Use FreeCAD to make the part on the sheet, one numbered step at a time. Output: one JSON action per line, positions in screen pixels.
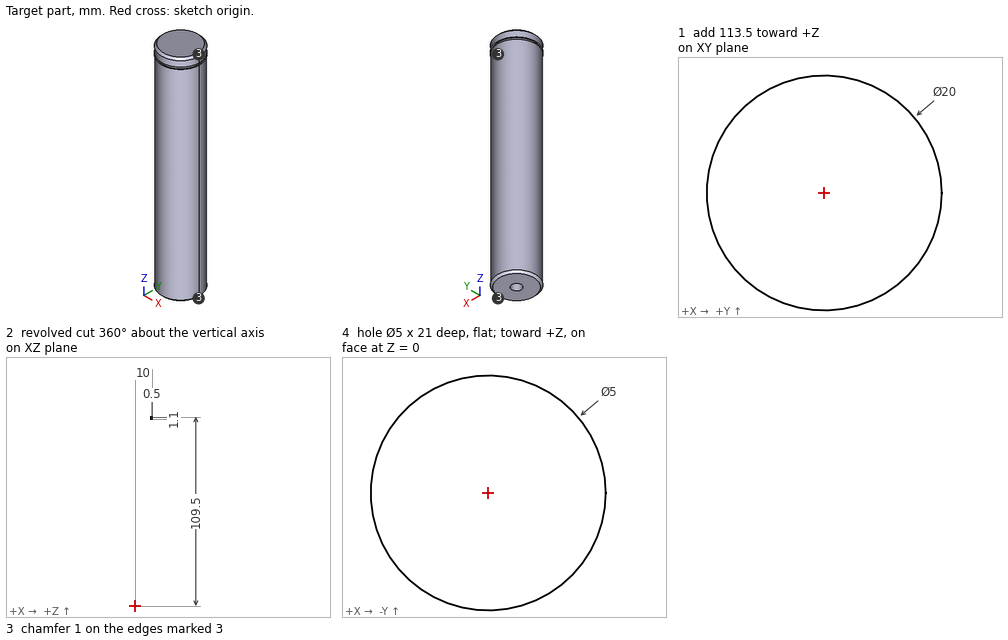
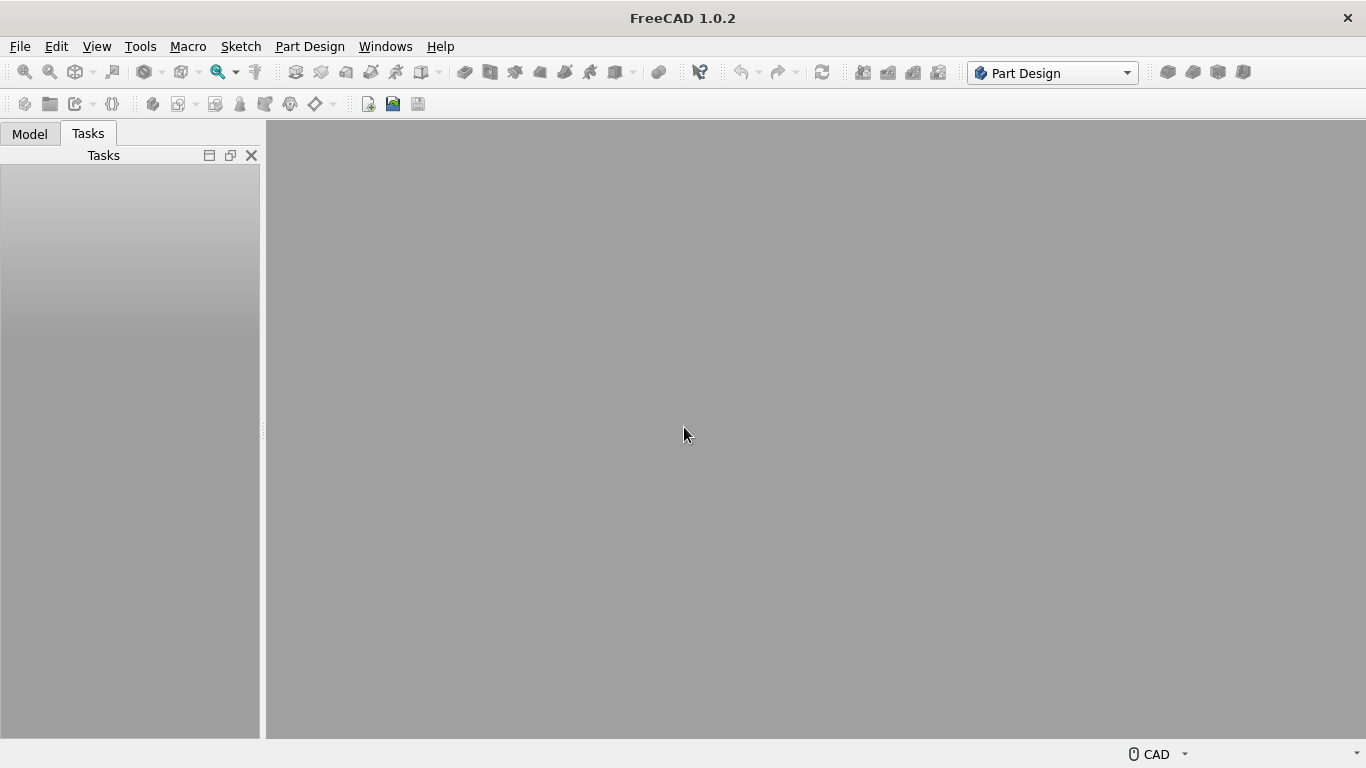
{"action": "key", "text": "ctrl+n"}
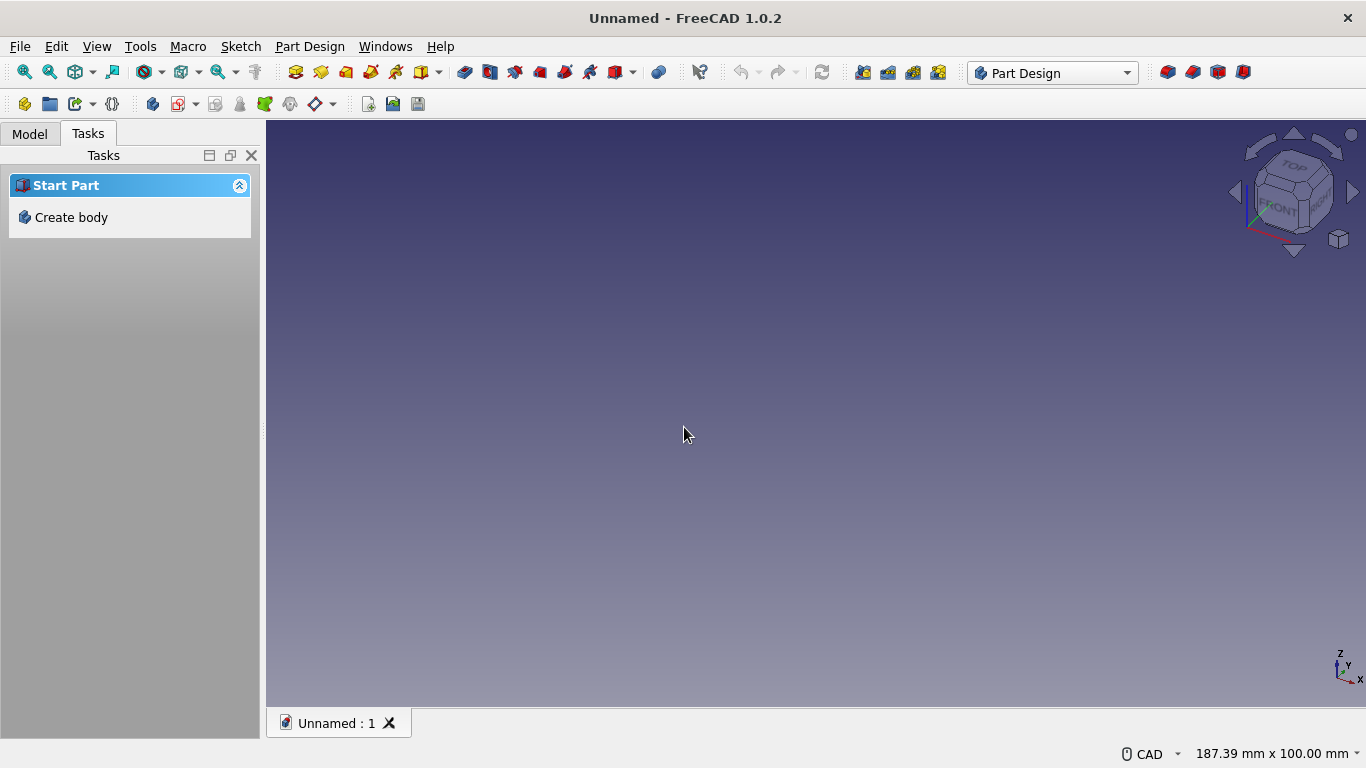
{"action": "left_click", "coordinate": [178, 104]}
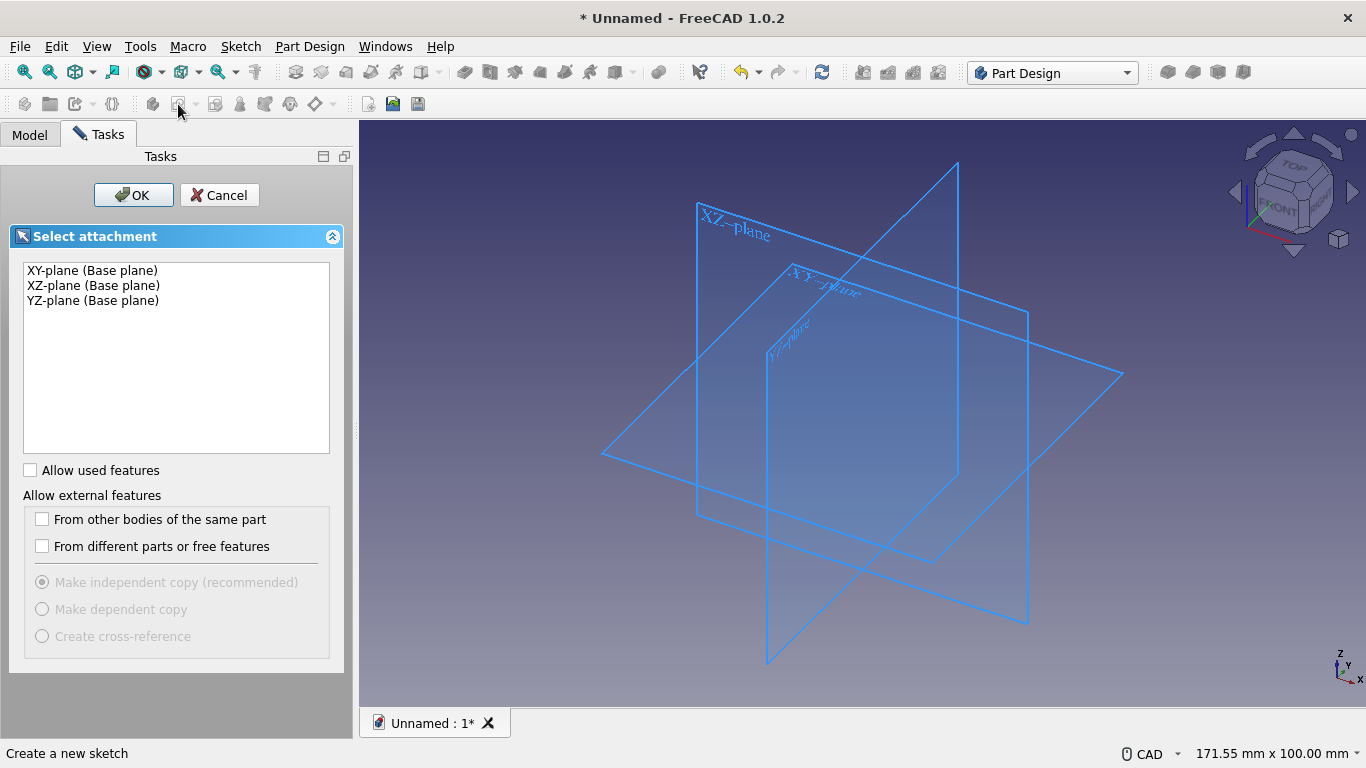
{"action": "left_click", "coordinate": [84, 270]}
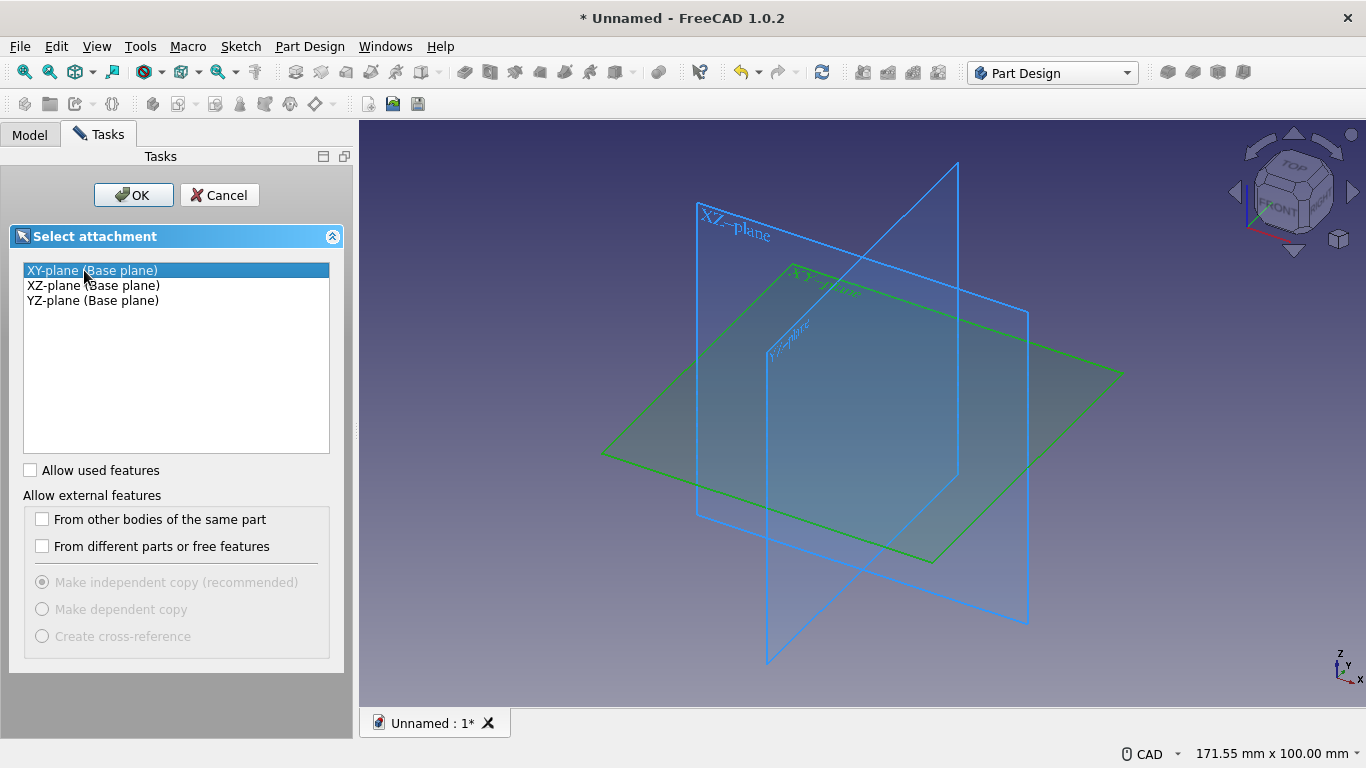
{"action": "left_click", "coordinate": [134, 195]}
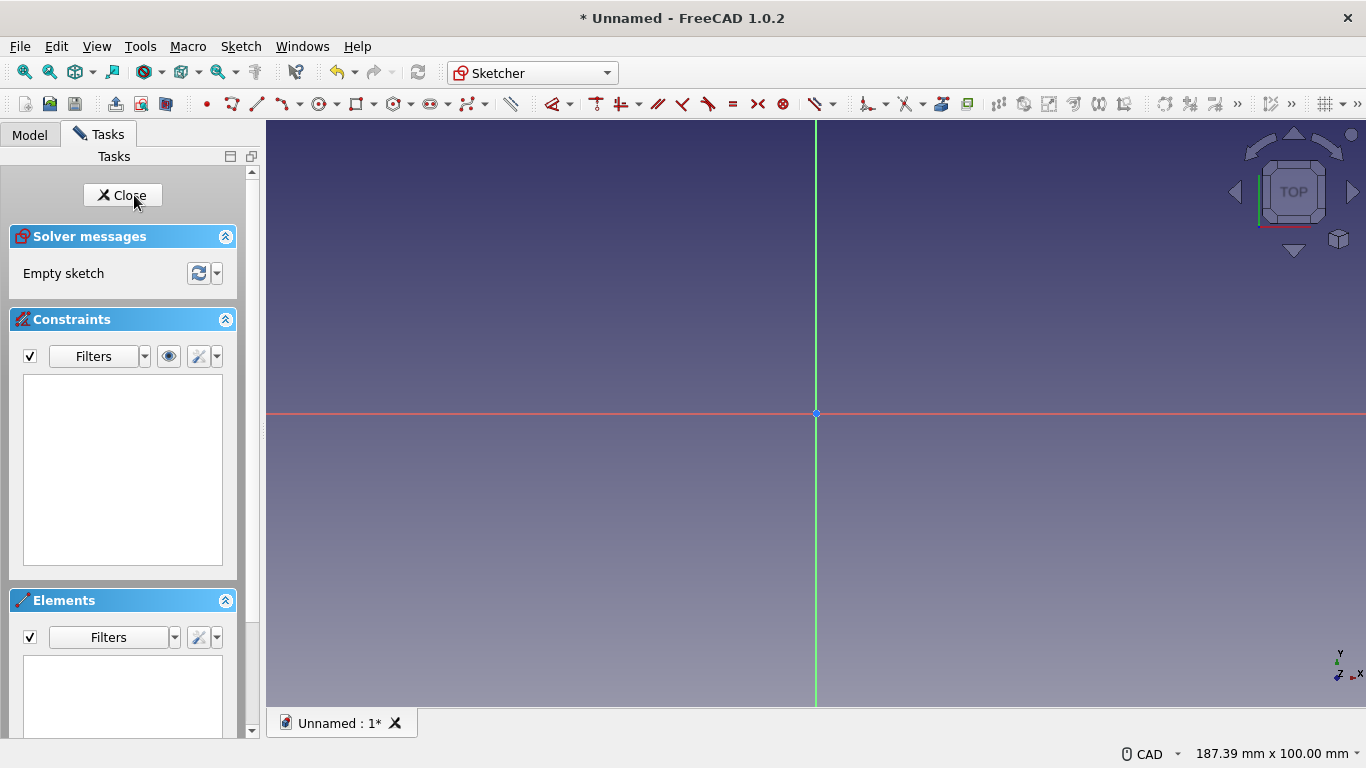
{"action": "scroll", "coordinate": [846, 414], "scroll_direction": "up", "scroll_amount": 6}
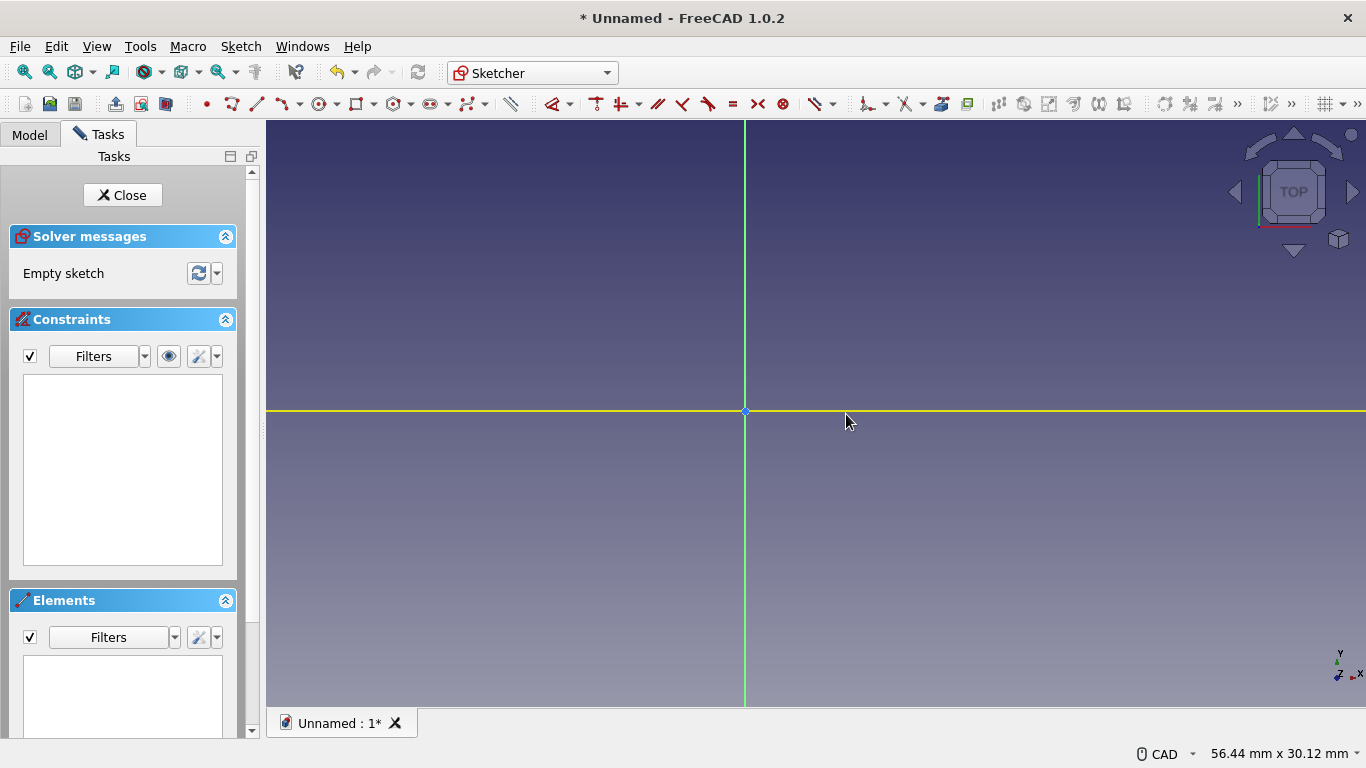
{"action": "key", "text": "g c"}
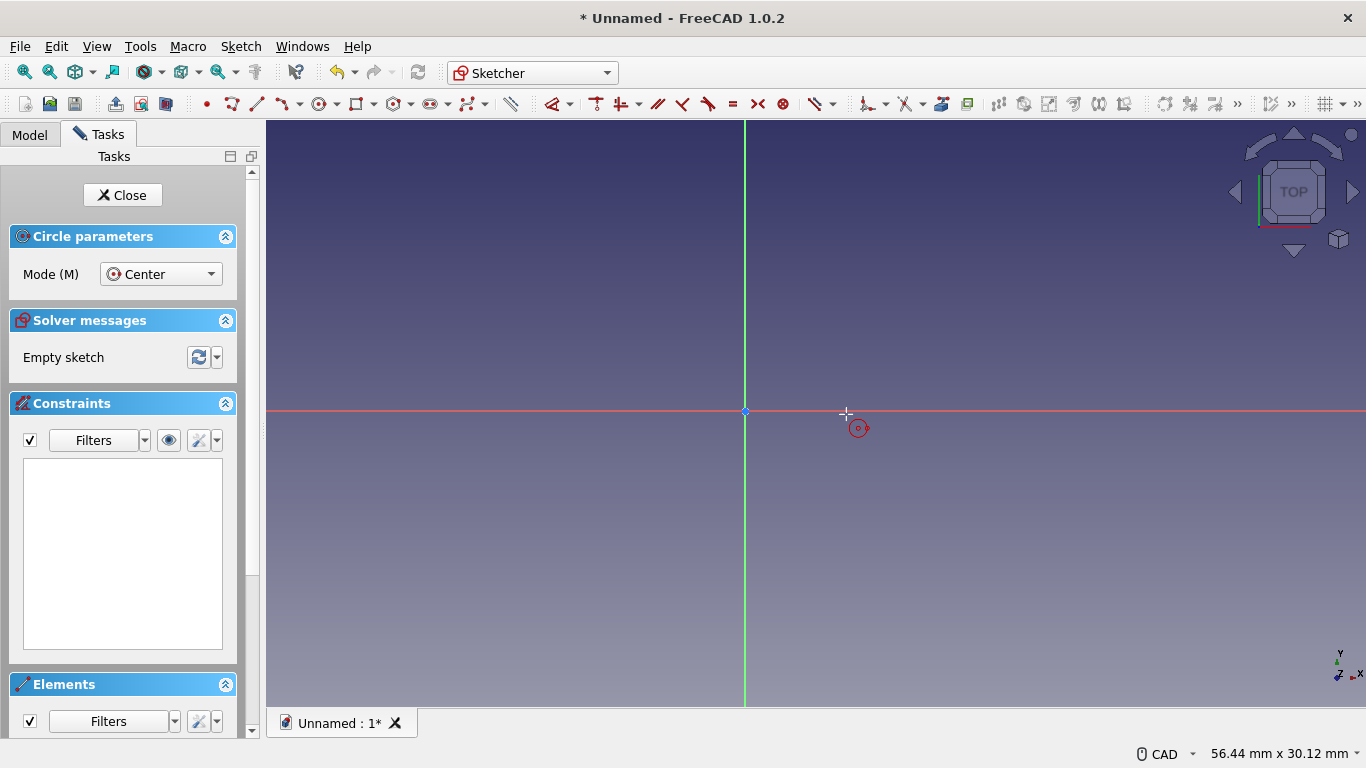
{"action": "left_click", "coordinate": [745, 411]}
{"action": "left_click", "coordinate": [883, 273]}
{"action": "key", "text": "Escape"}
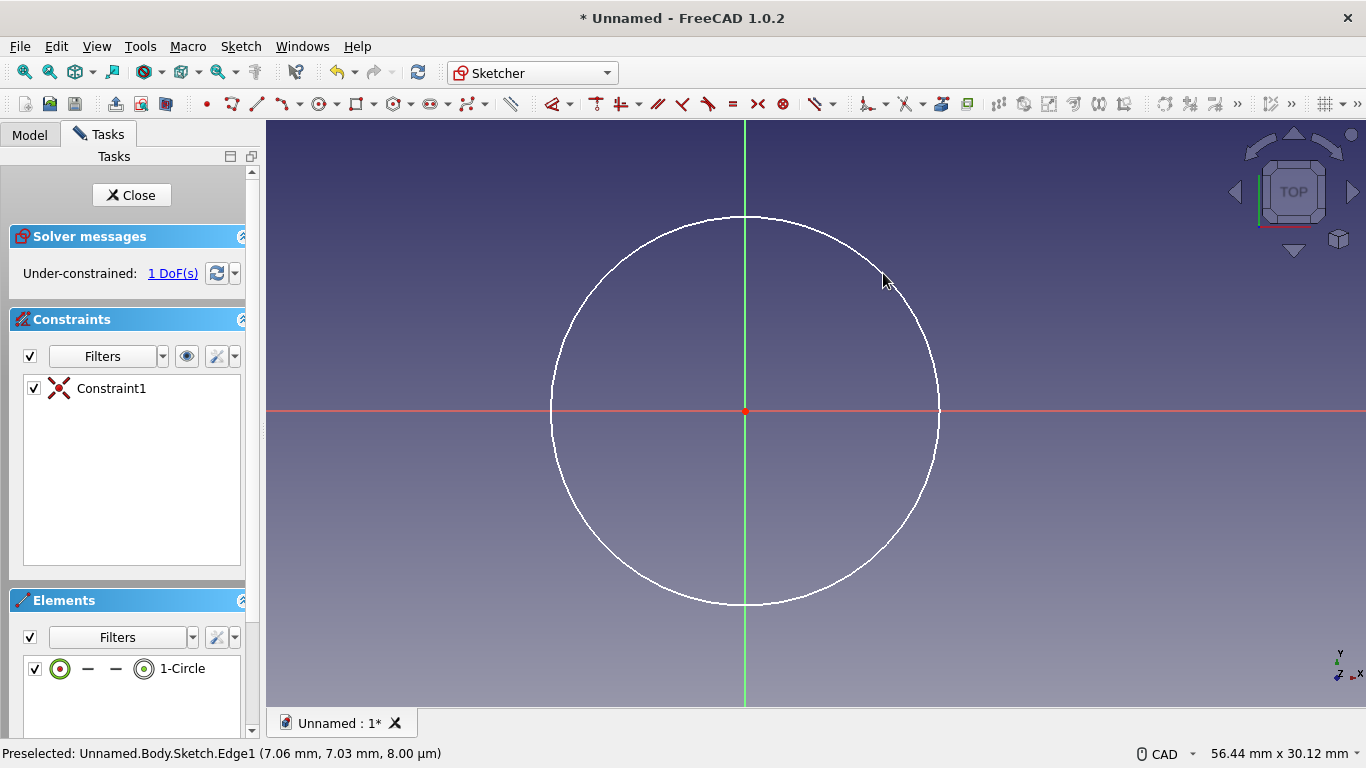
{"action": "left_click", "coordinate": [552, 104]}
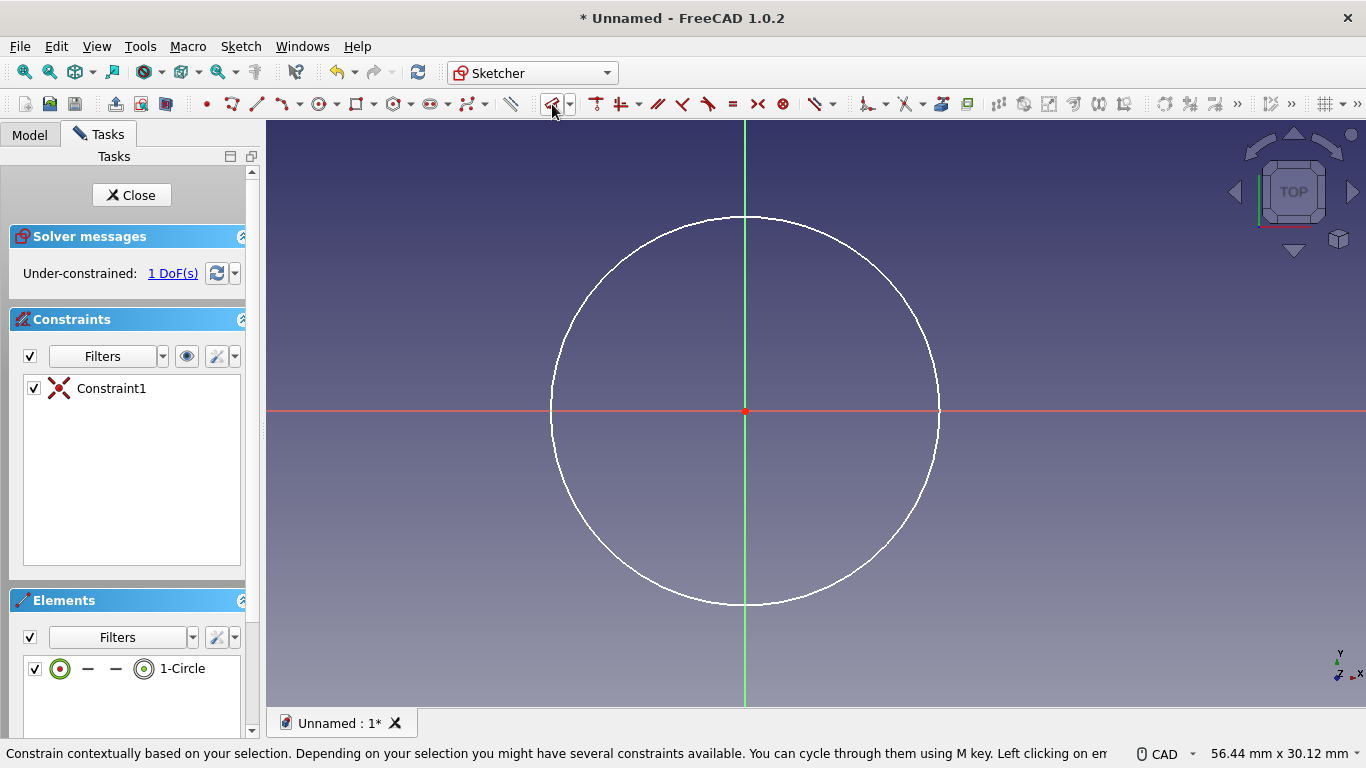
{"action": "left_click", "coordinate": [882, 273]}
{"action": "left_click", "coordinate": [905, 250]}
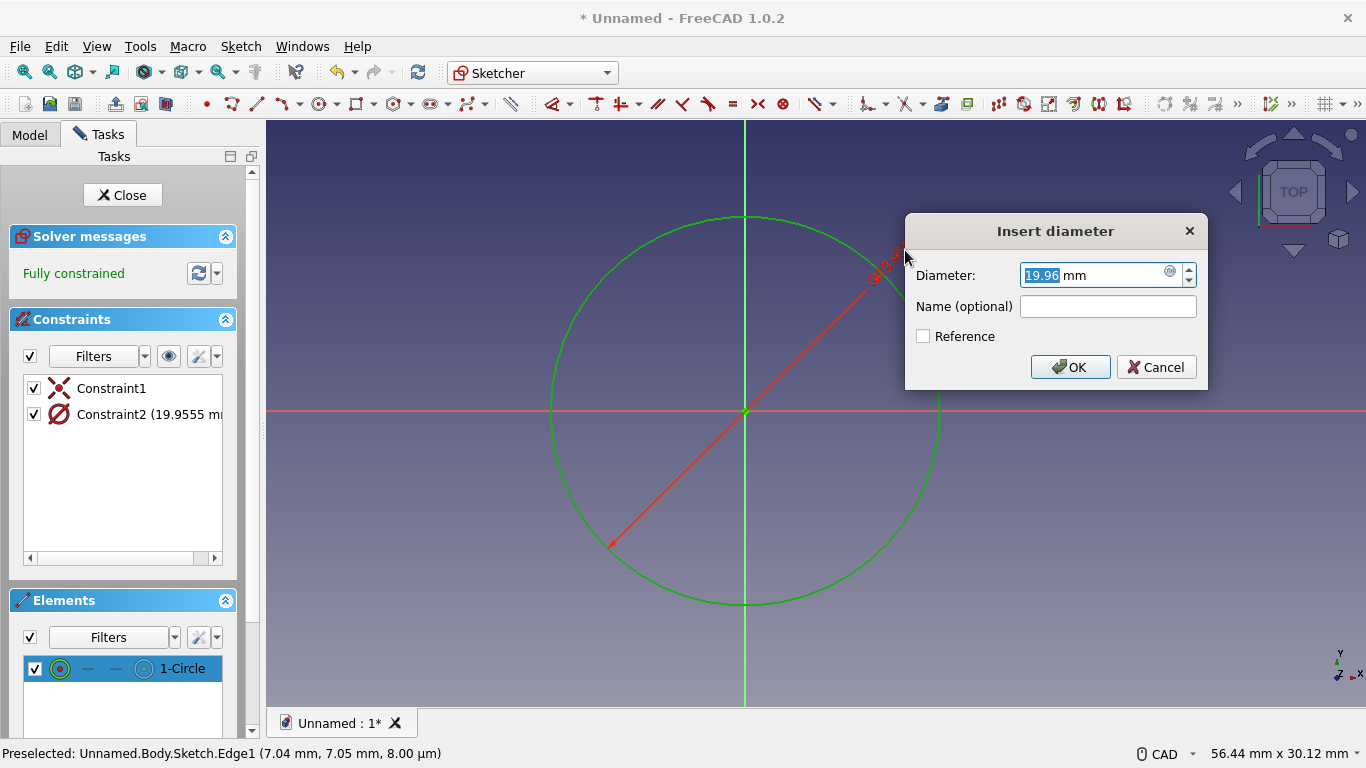
{"action": "type", "text": "20"}
{"action": "key", "text": "Return"}
{"action": "key", "text": "Escape"}